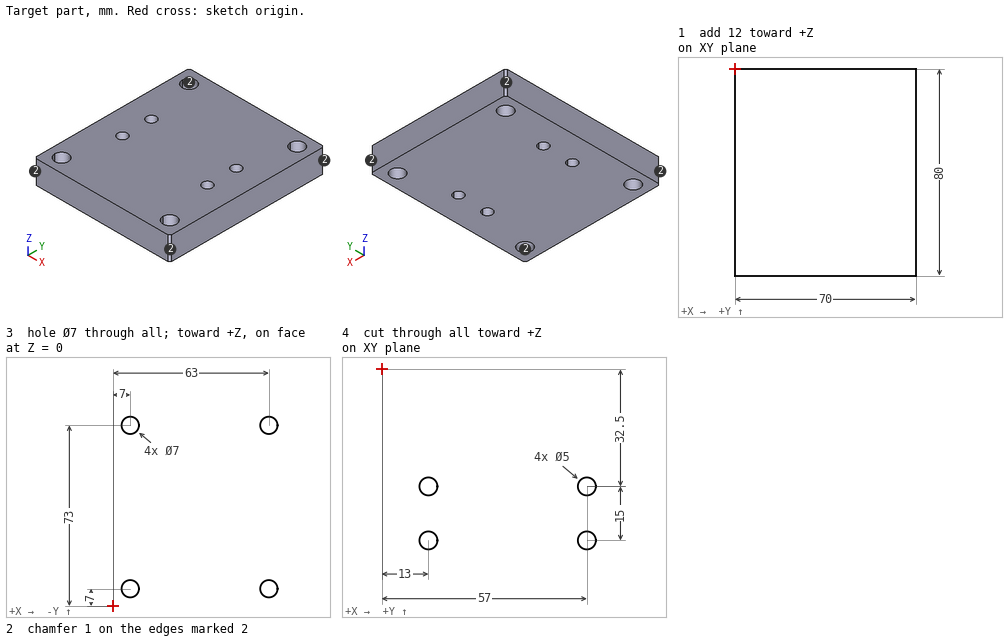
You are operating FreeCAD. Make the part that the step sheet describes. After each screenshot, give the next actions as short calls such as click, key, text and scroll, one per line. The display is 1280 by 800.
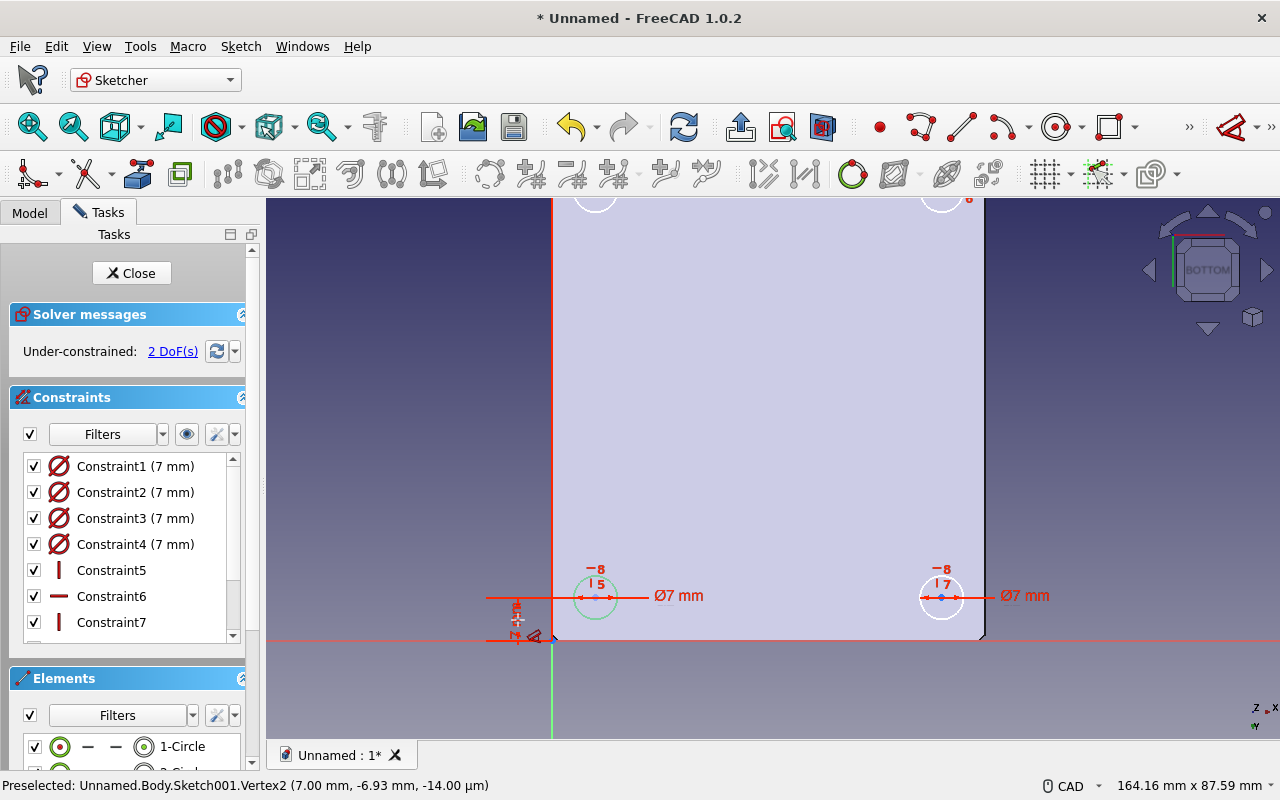
scroll(596, 598, down, 2)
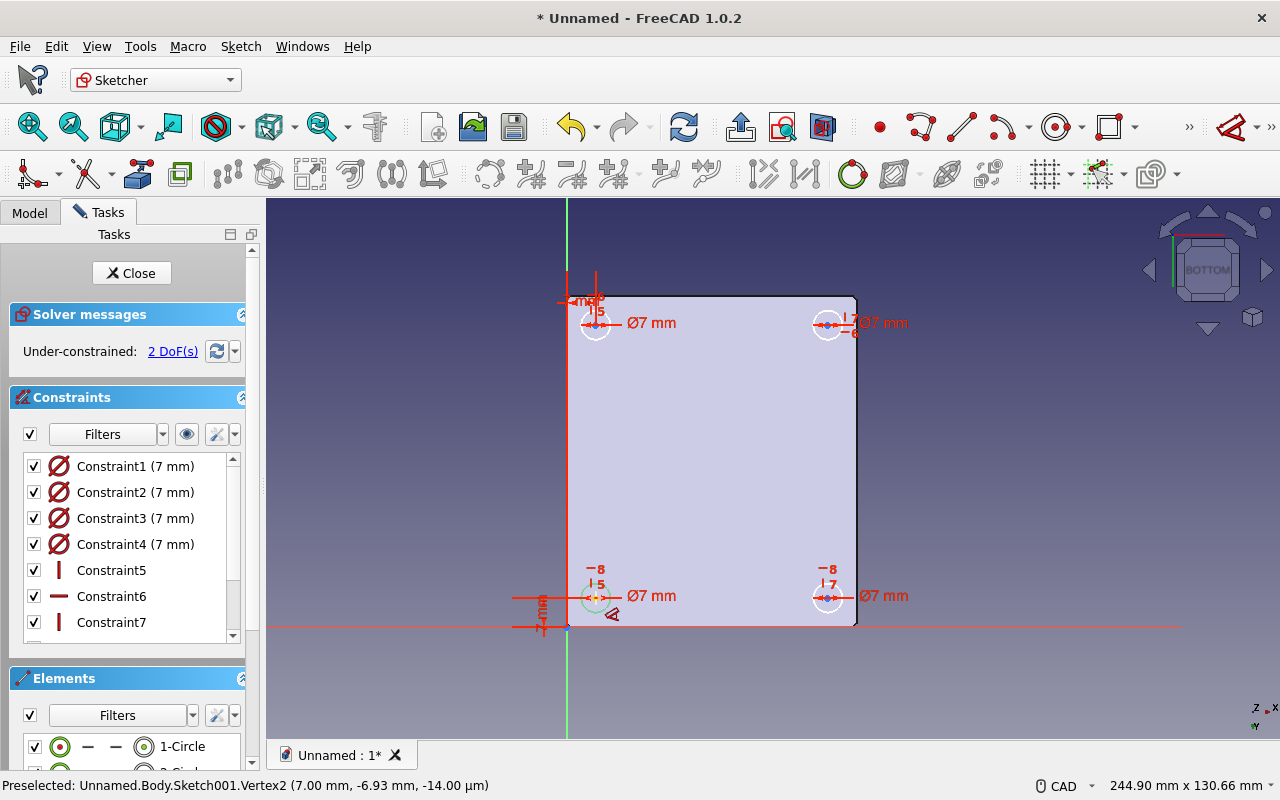
click(596, 325)
click(533, 476)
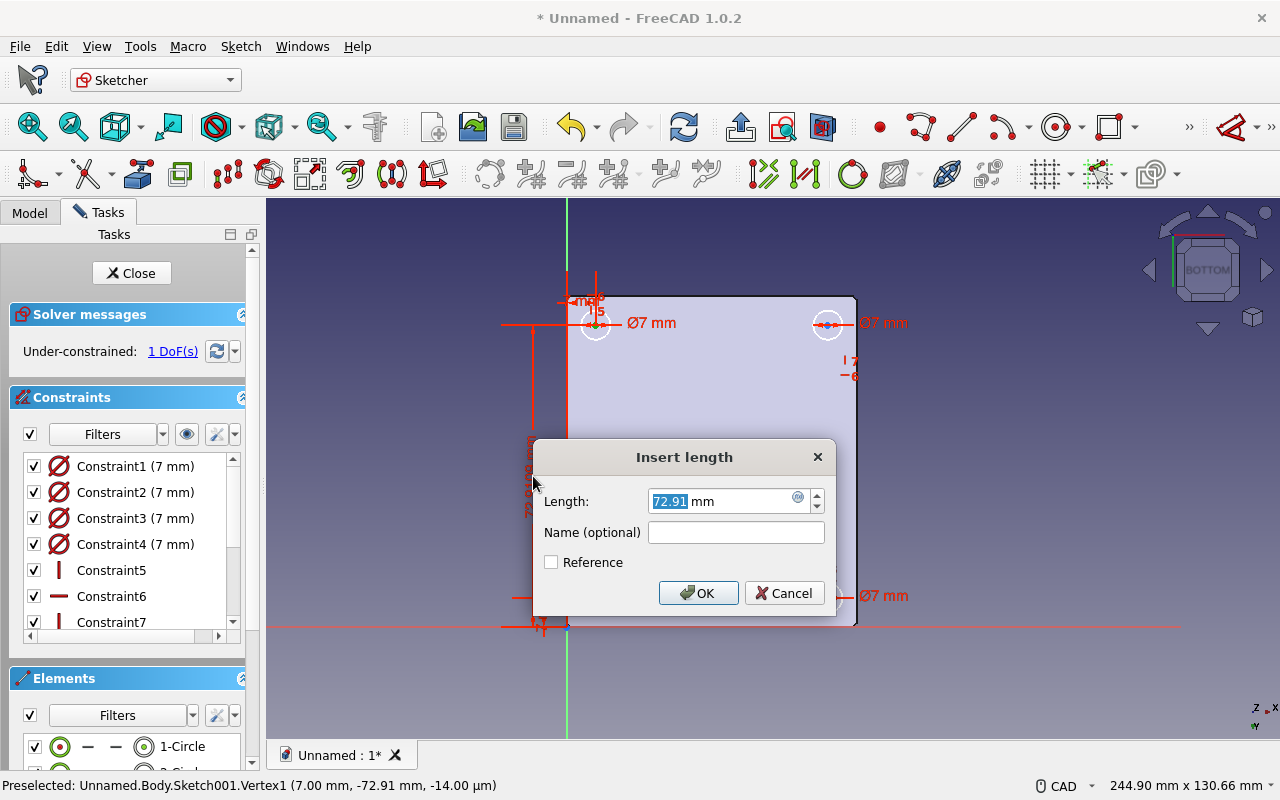
text(73)
key(Return)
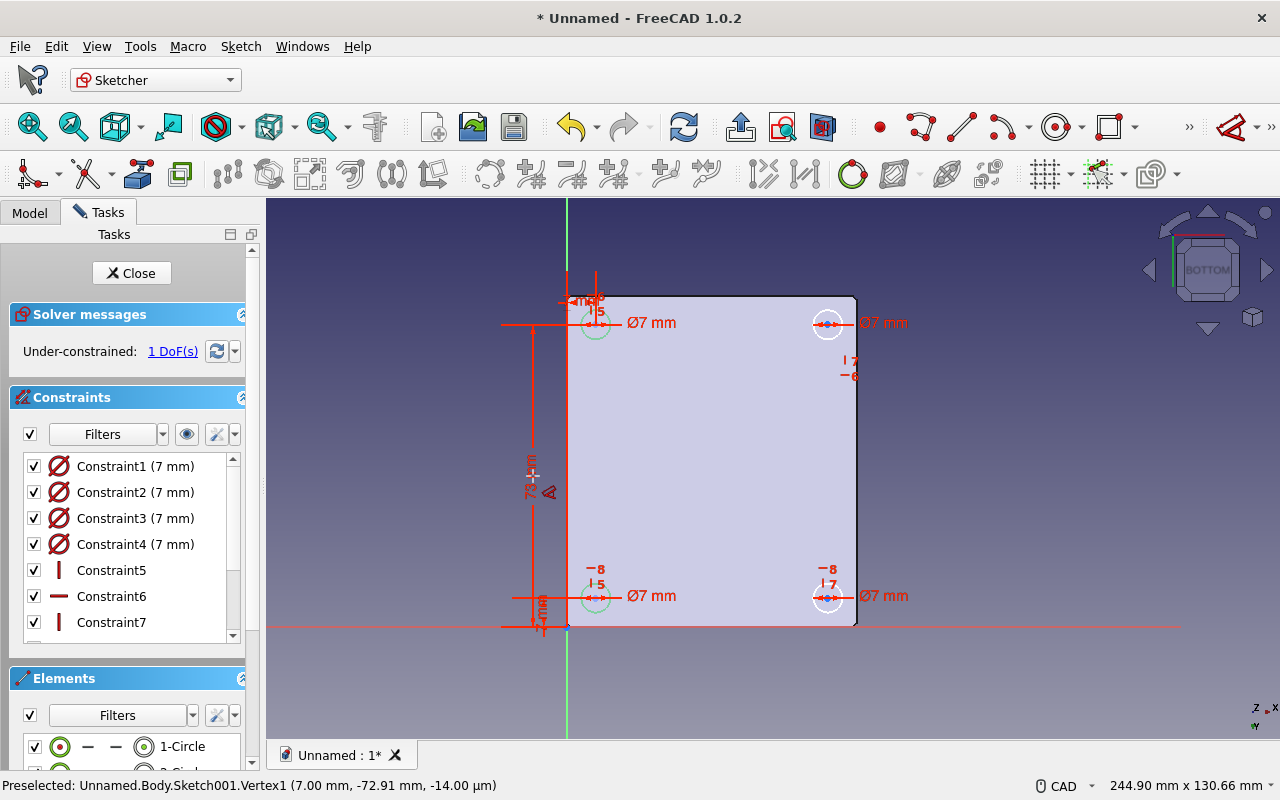
click(828, 325)
click(697, 661)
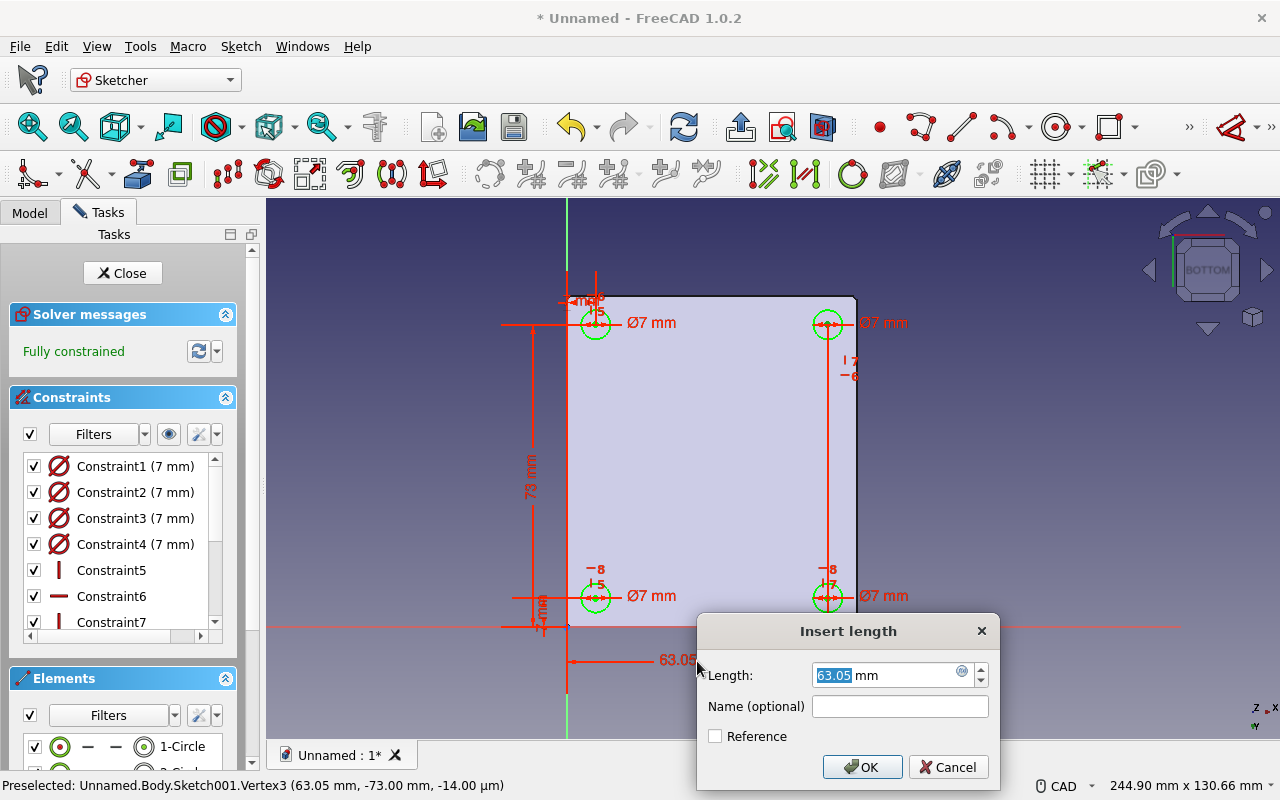
text(63)
key(Return)
key(Escape)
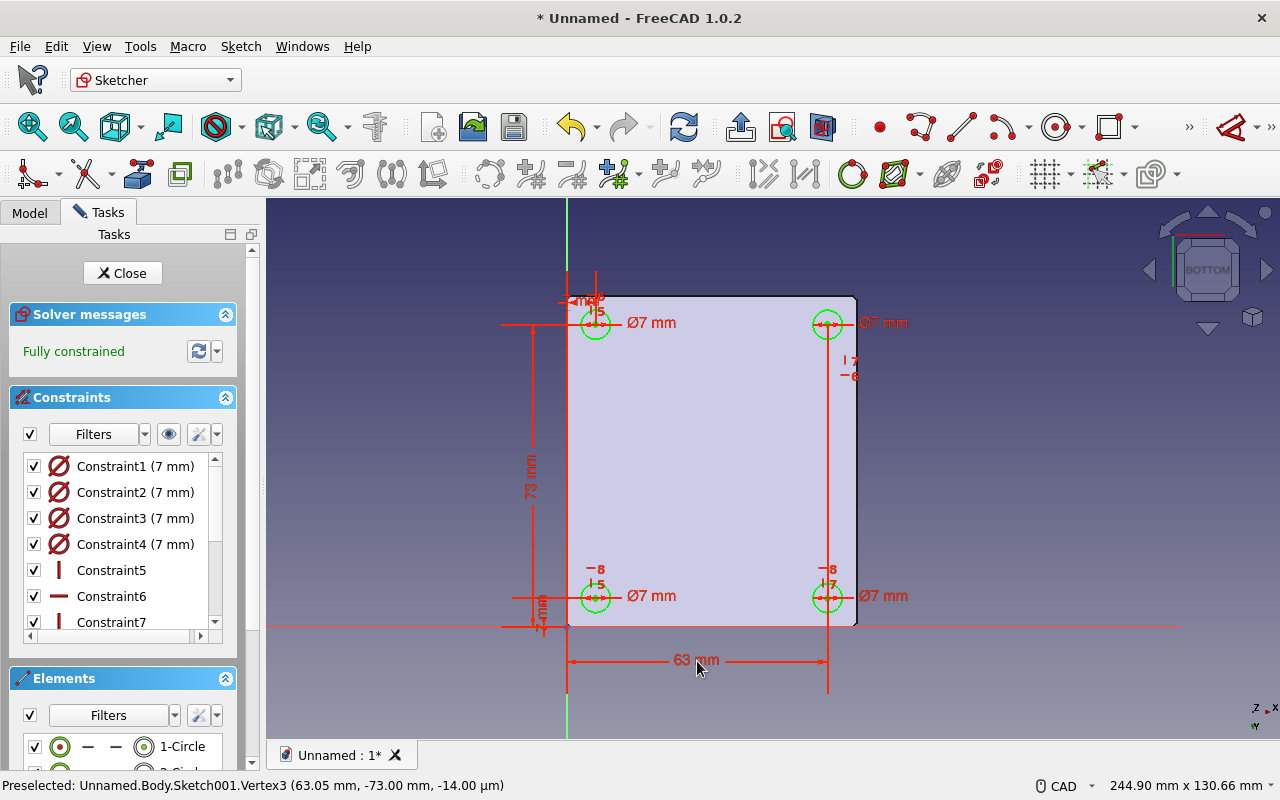
click(123, 273)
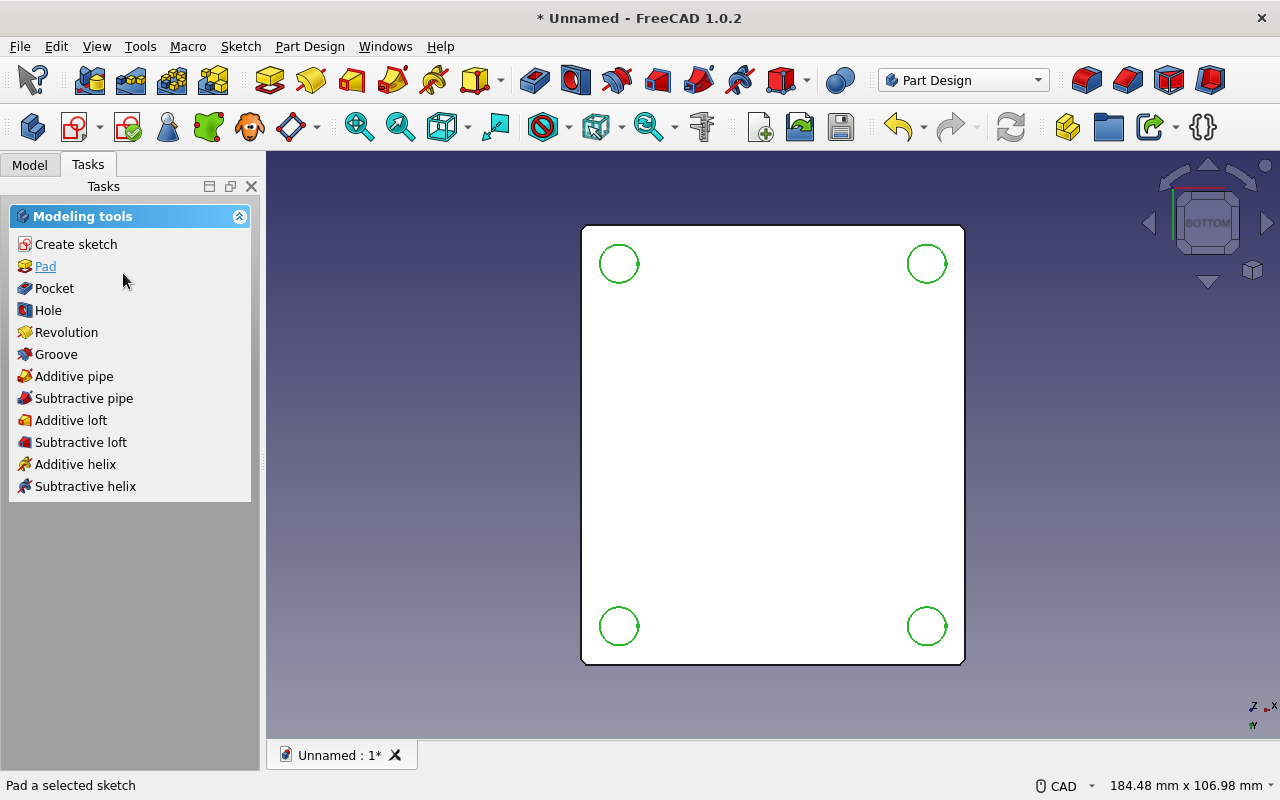
click(576, 80)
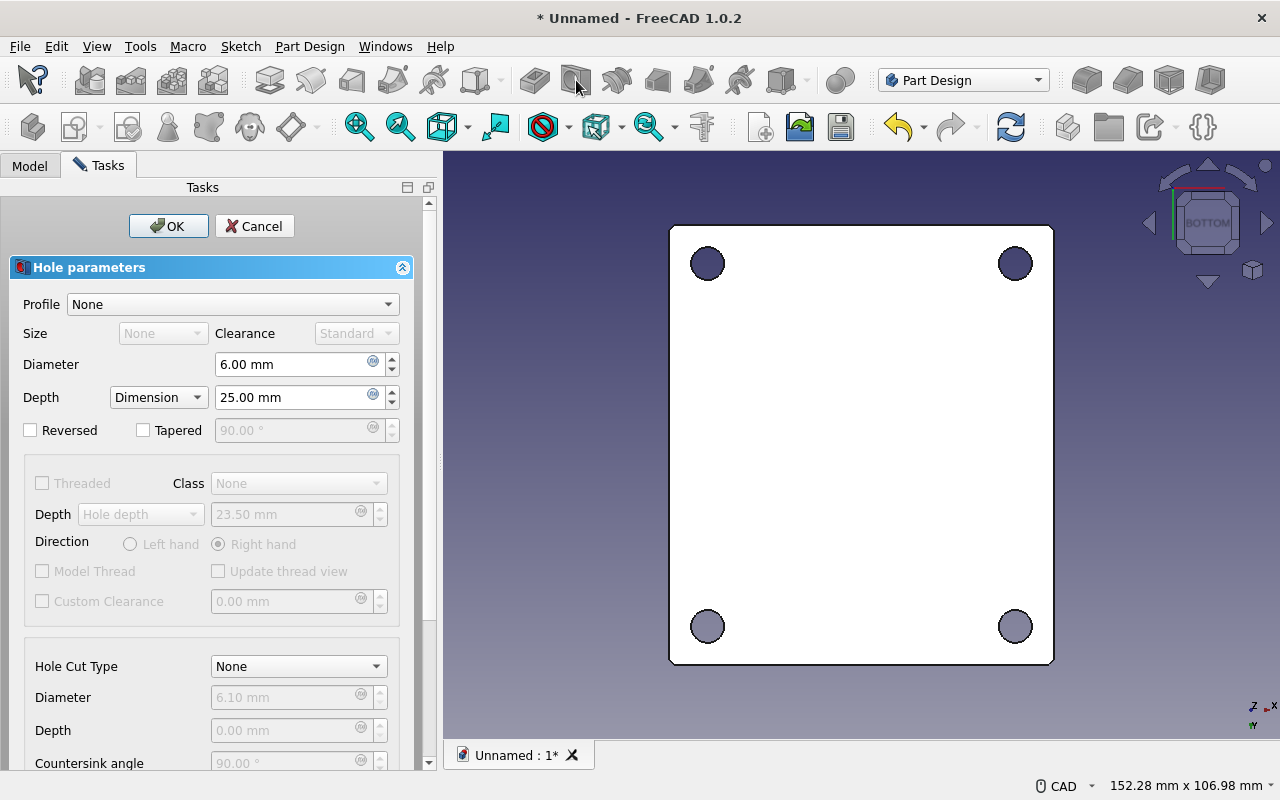
triple_click(300, 364)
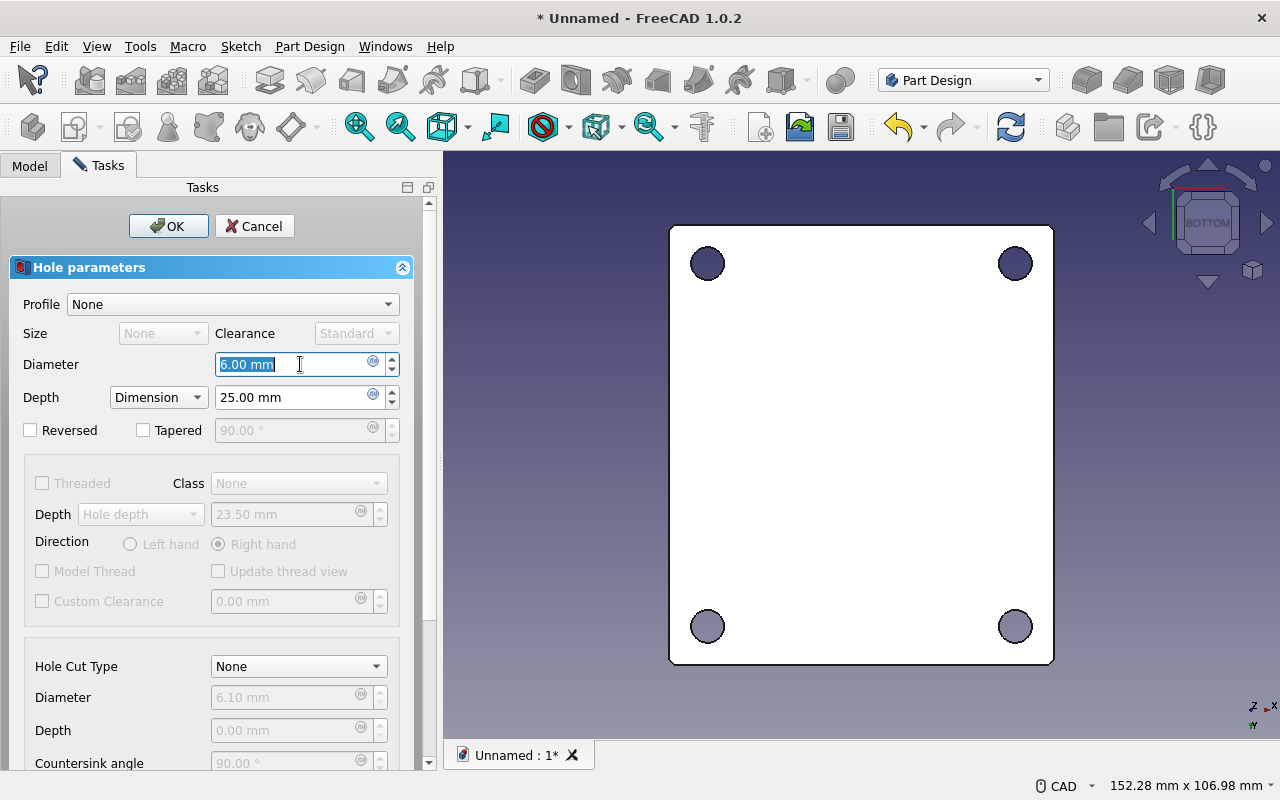
text(7)
key(Tab)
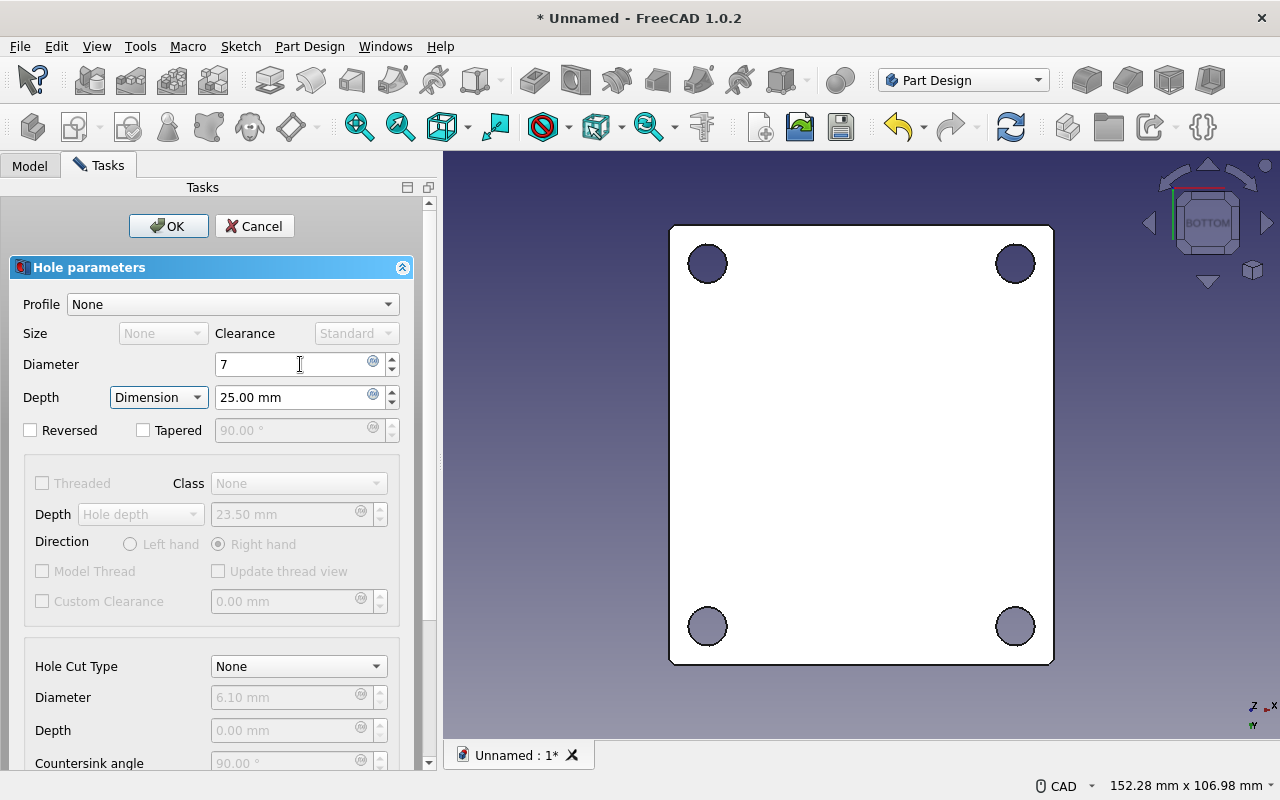
click(160, 398)